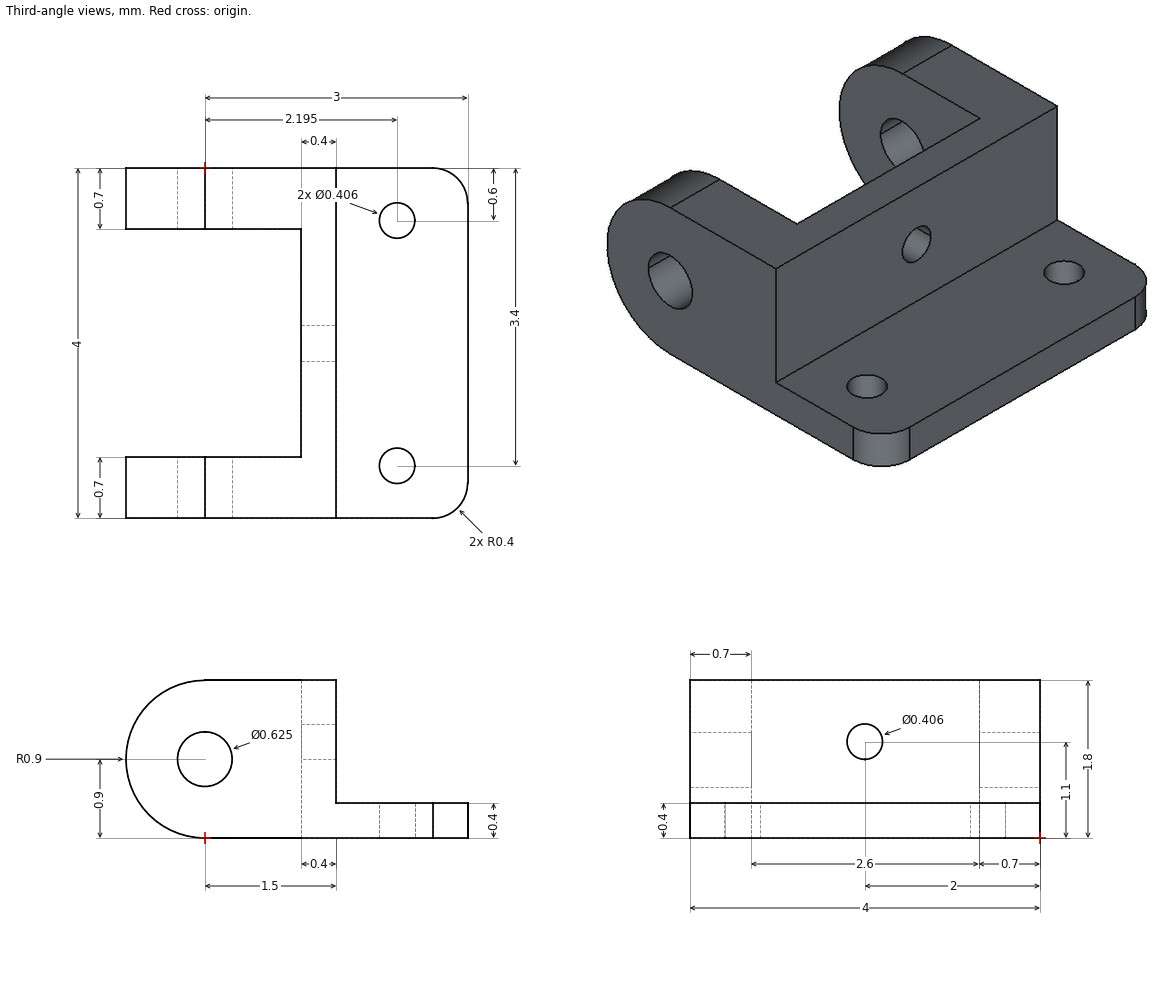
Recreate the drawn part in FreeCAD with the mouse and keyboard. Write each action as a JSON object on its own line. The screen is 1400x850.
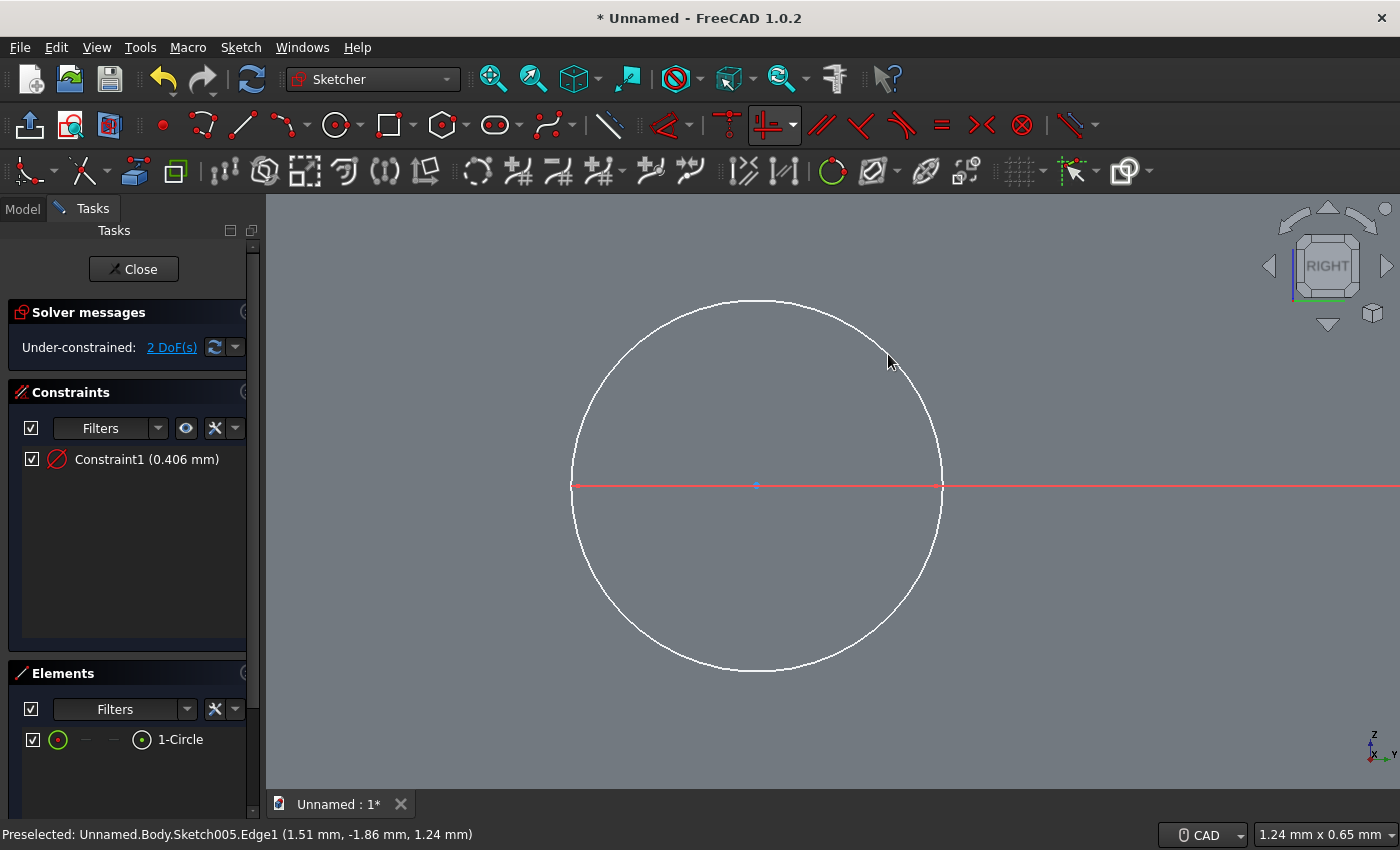
{"action": "key", "text": "d"}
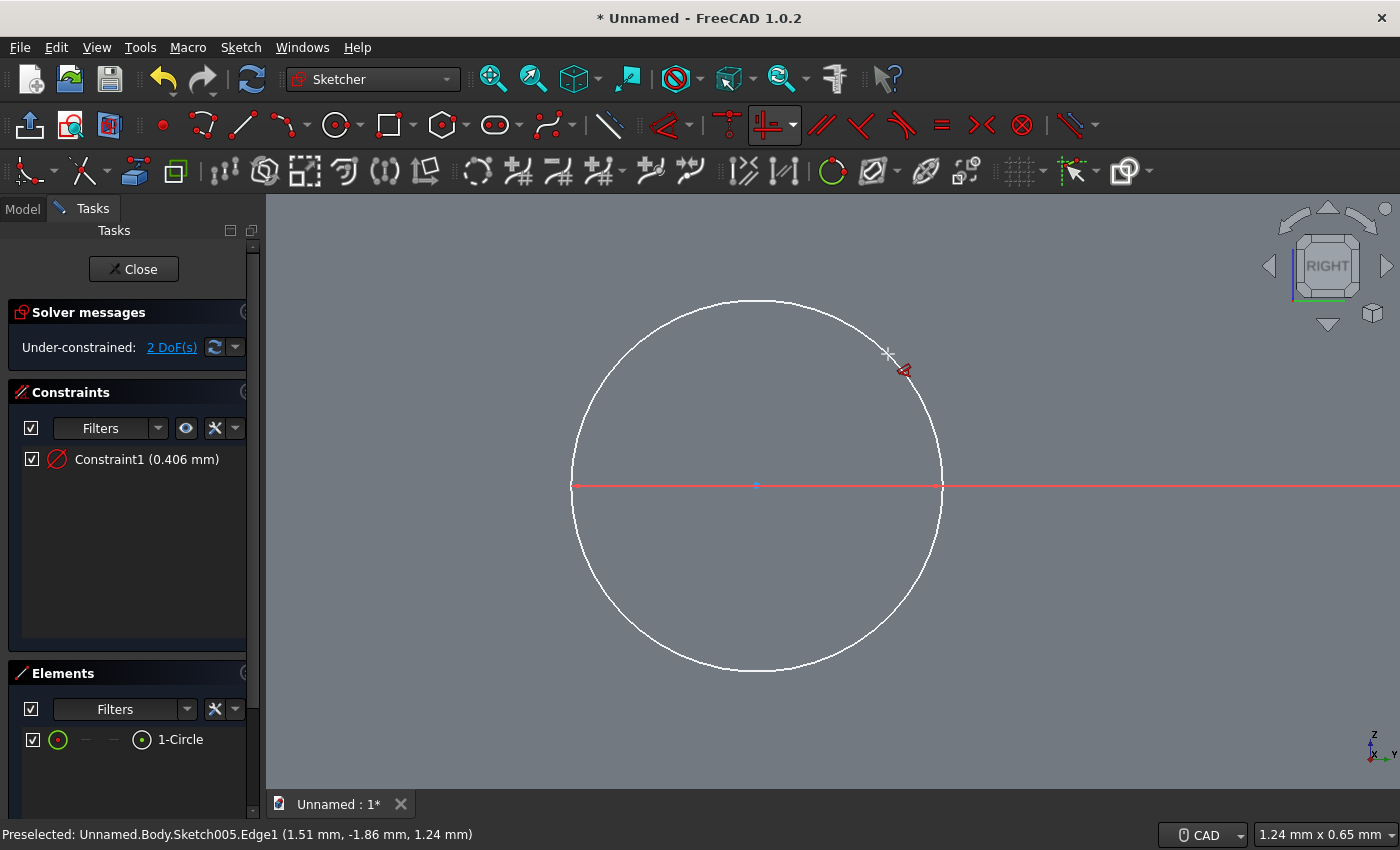
{"action": "left_click", "coordinate": [757, 486]}
{"action": "left_click", "coordinate": [996, 452]}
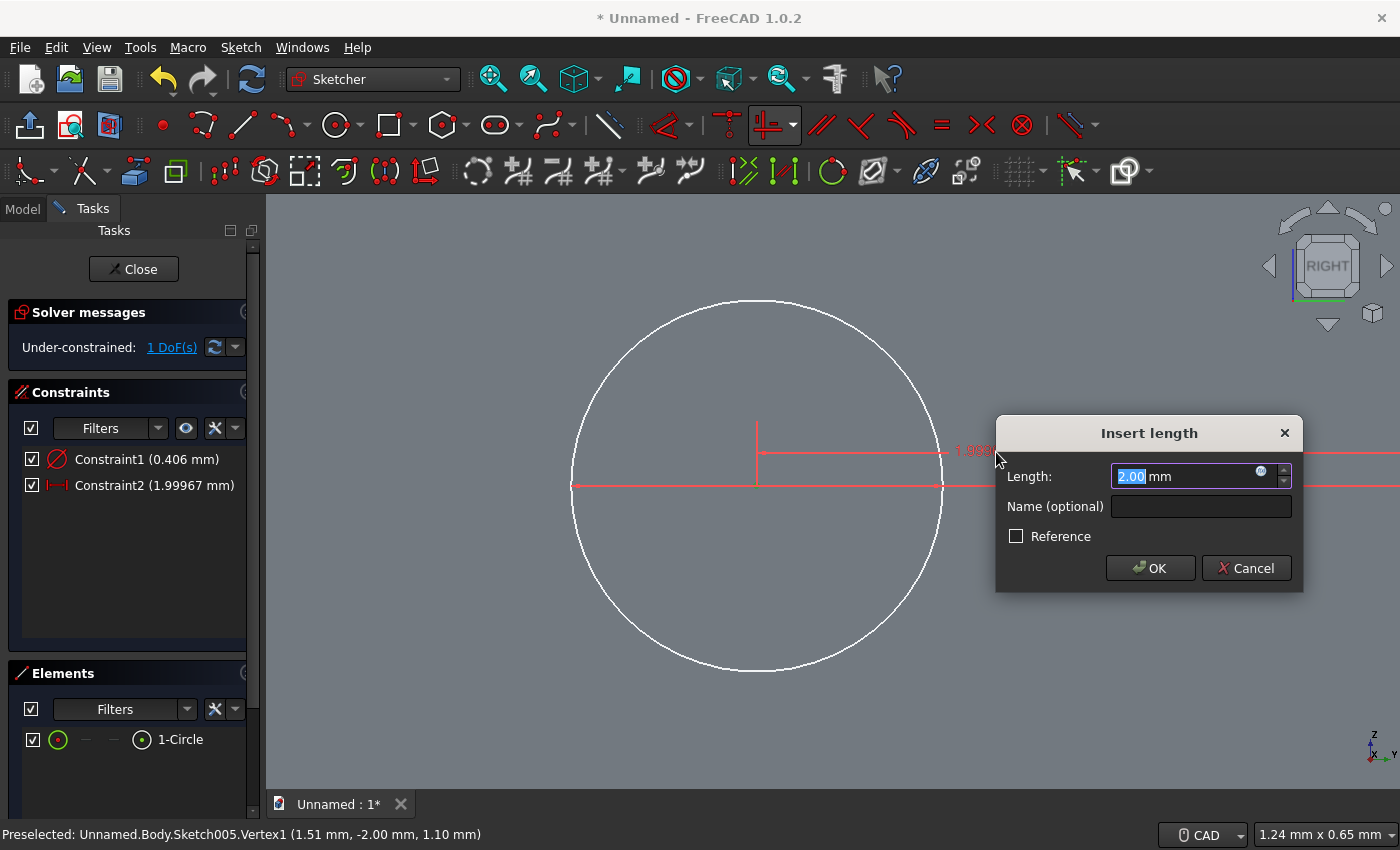
{"action": "type", "text": "2"}
{"action": "key", "text": "Return"}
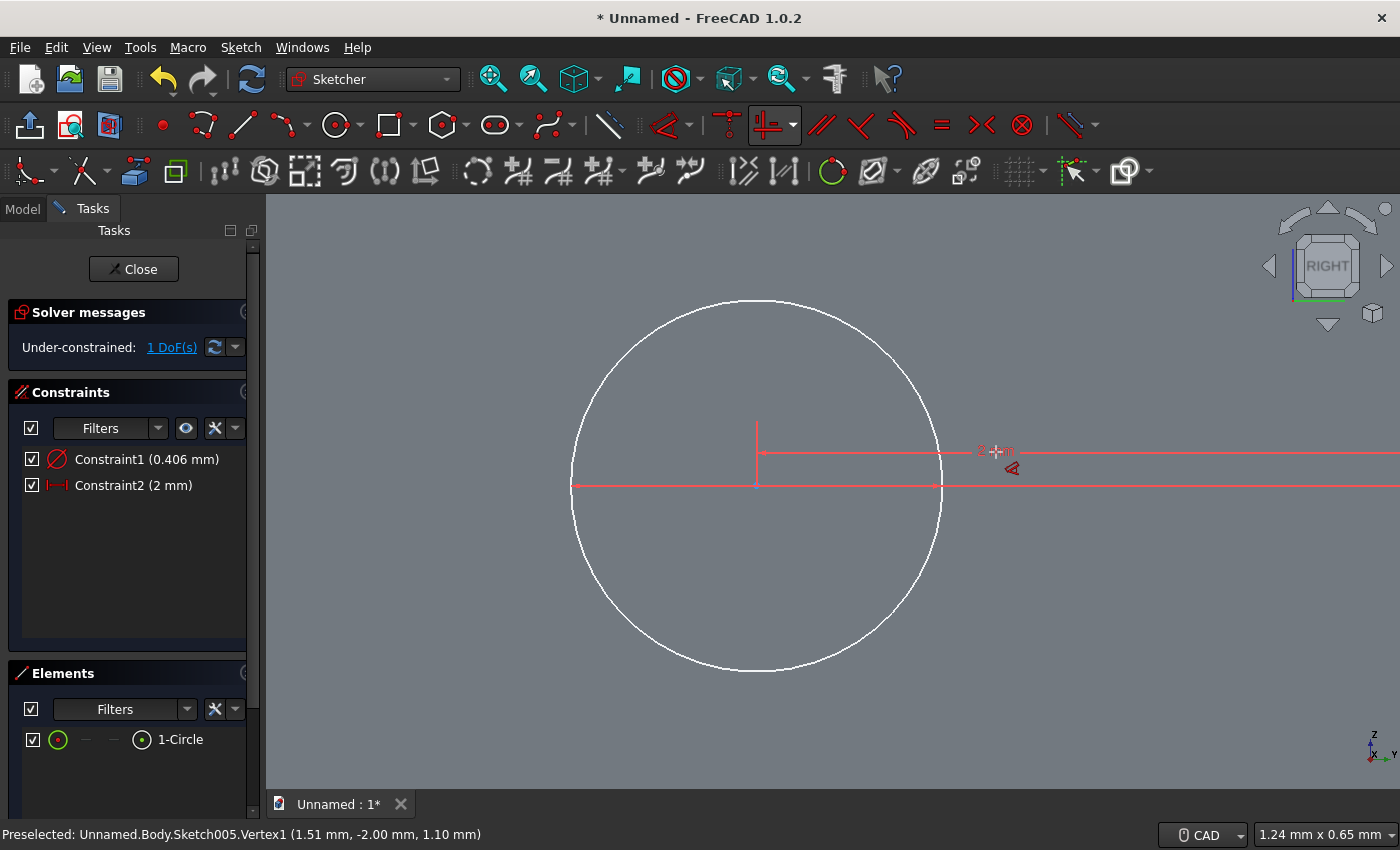
{"action": "left_click", "coordinate": [757, 486]}
{"action": "left_click", "coordinate": [723, 623]}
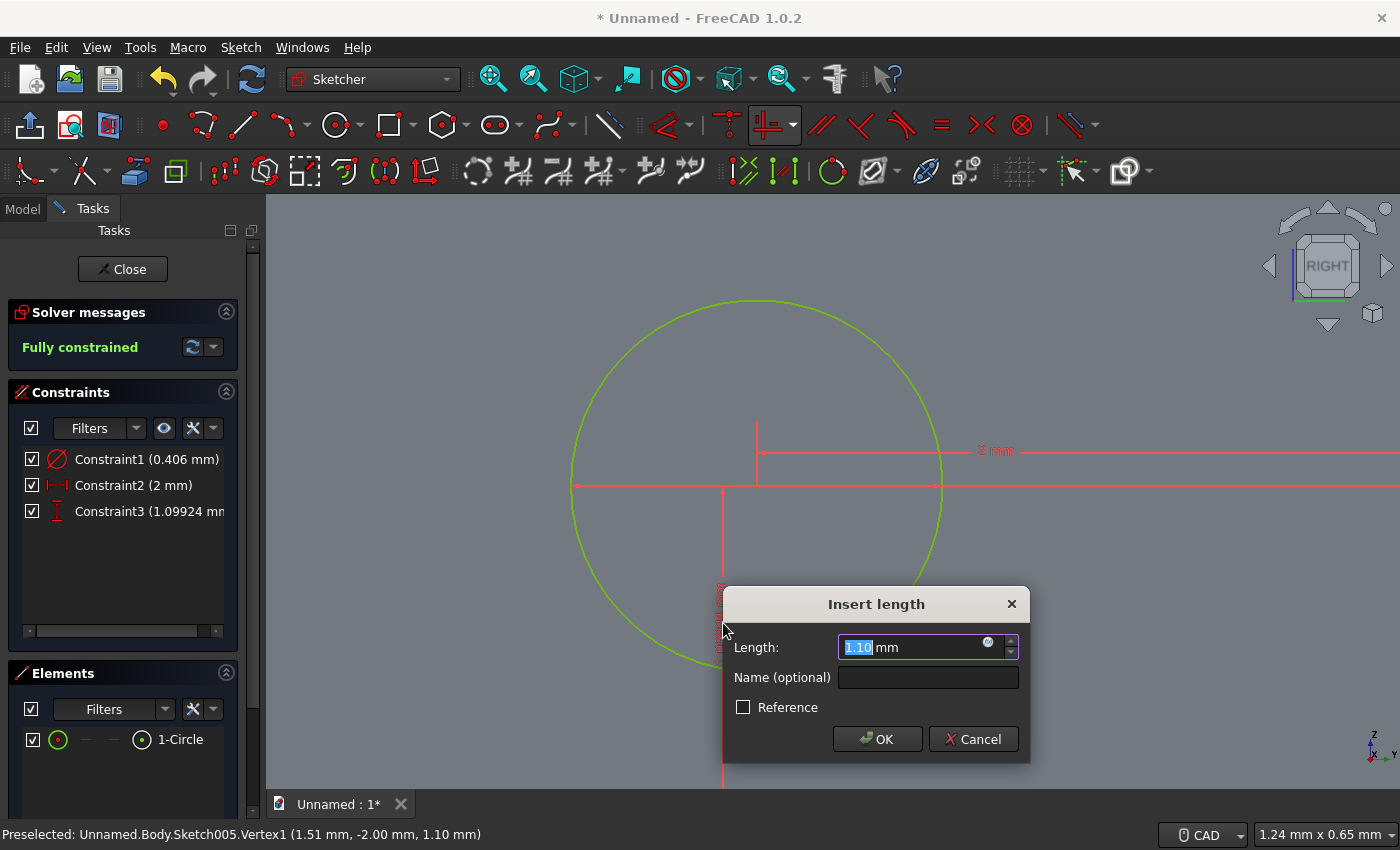
{"action": "type", "text": "1.1"}
{"action": "key", "text": "Return"}
{"action": "key", "text": "Escape"}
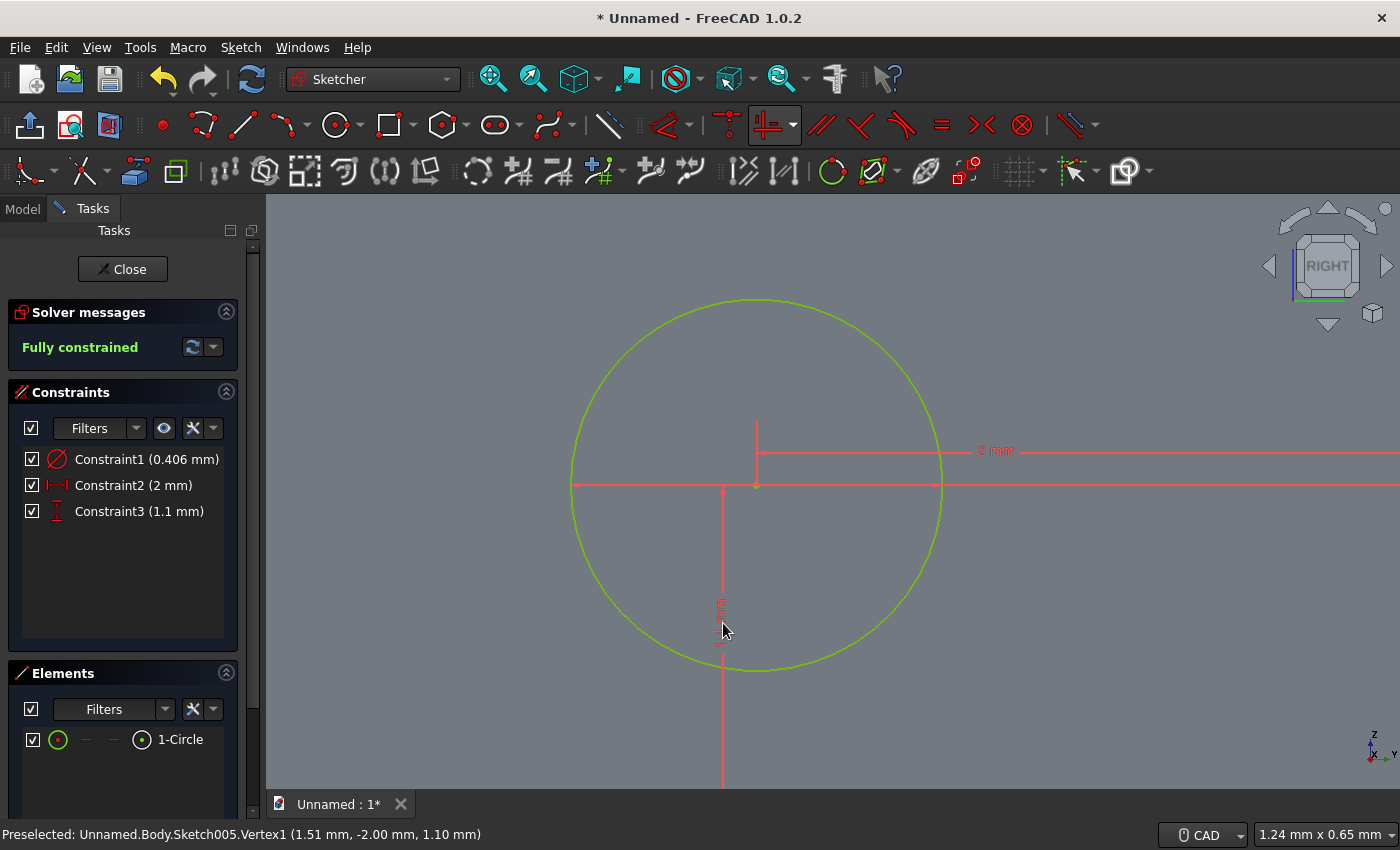
{"action": "left_click", "coordinate": [123, 269]}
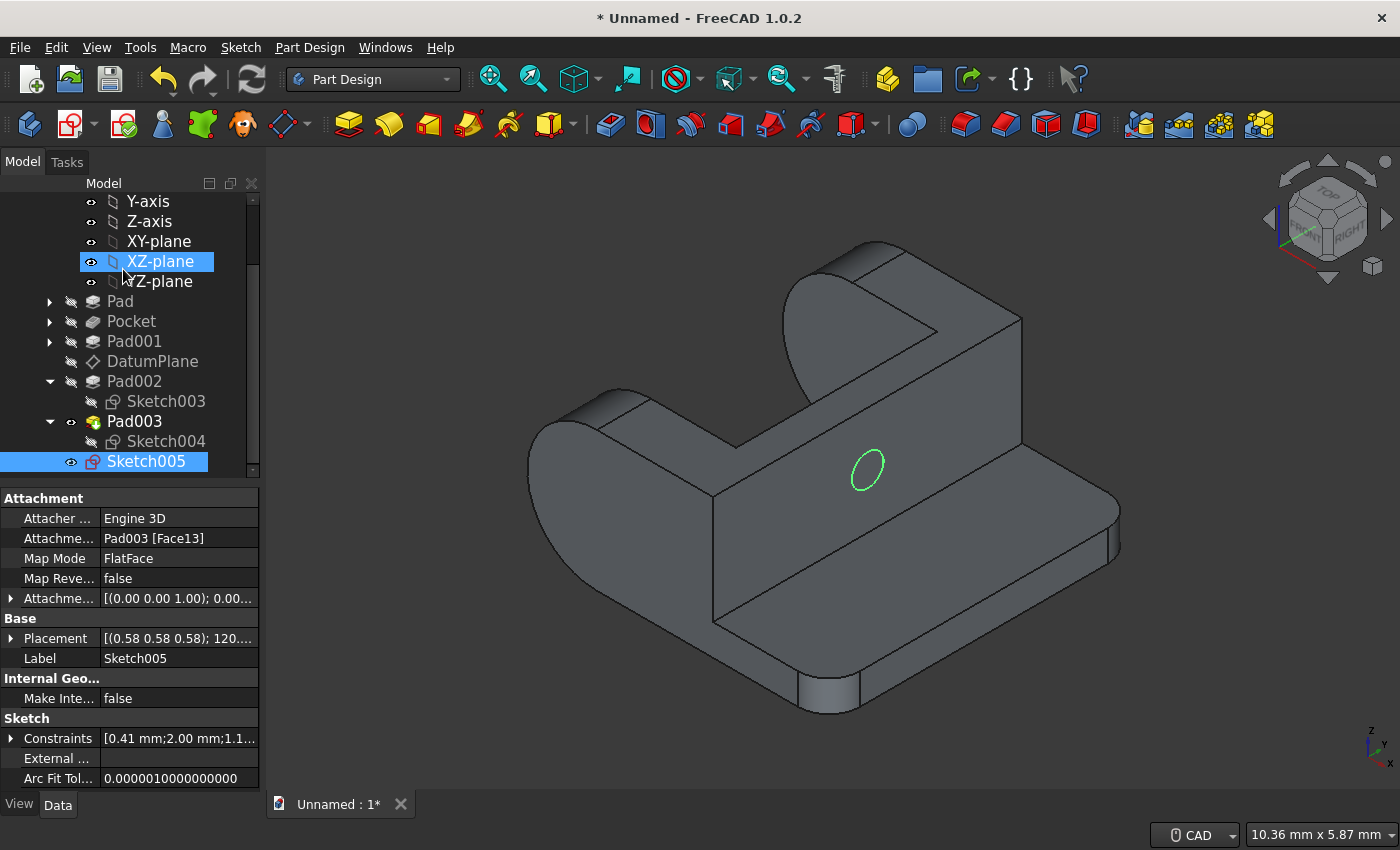
{"action": "left_click", "coordinate": [612, 124]}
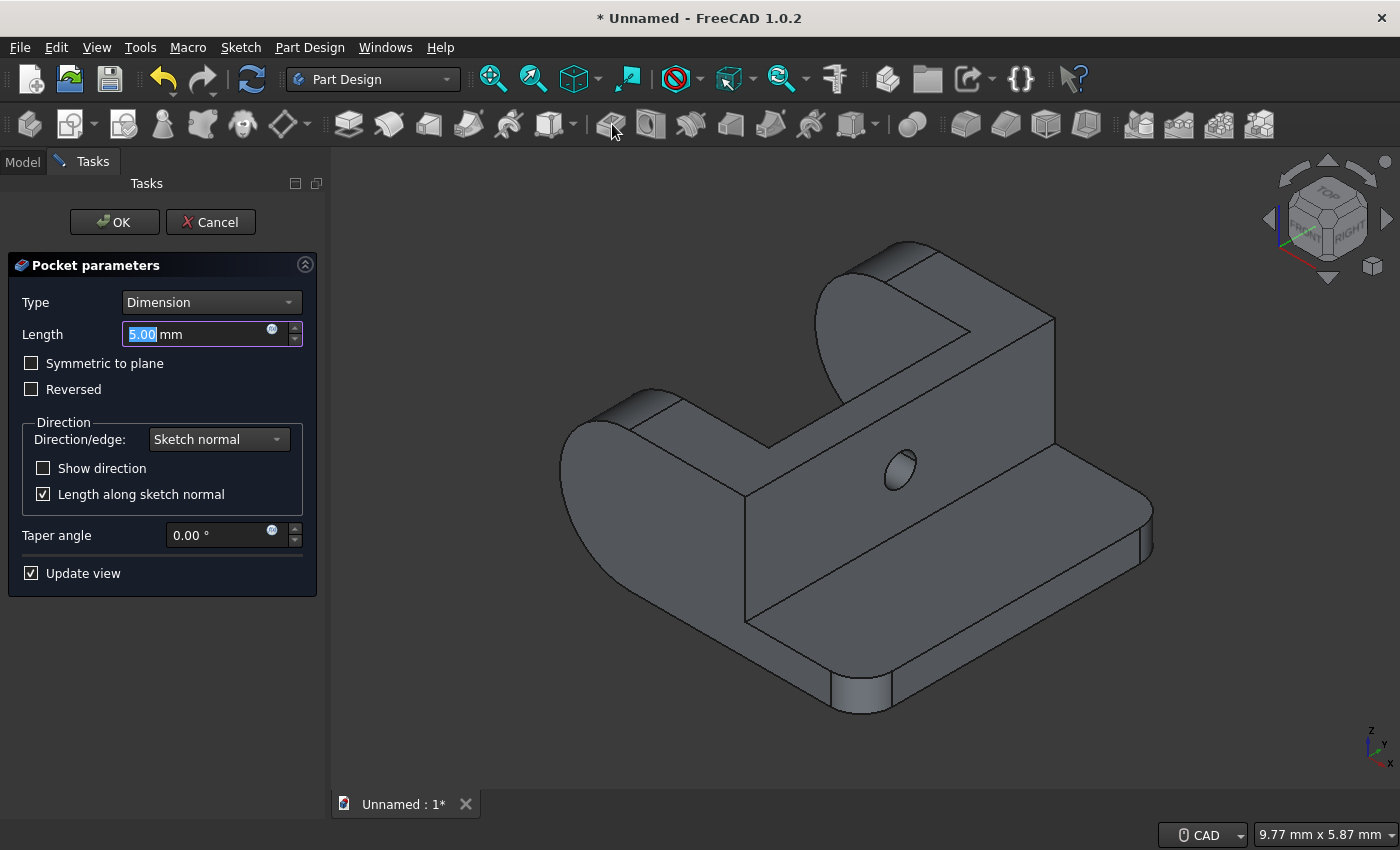
{"action": "type", "text": "0.4"}
{"action": "key", "text": "Tab"}